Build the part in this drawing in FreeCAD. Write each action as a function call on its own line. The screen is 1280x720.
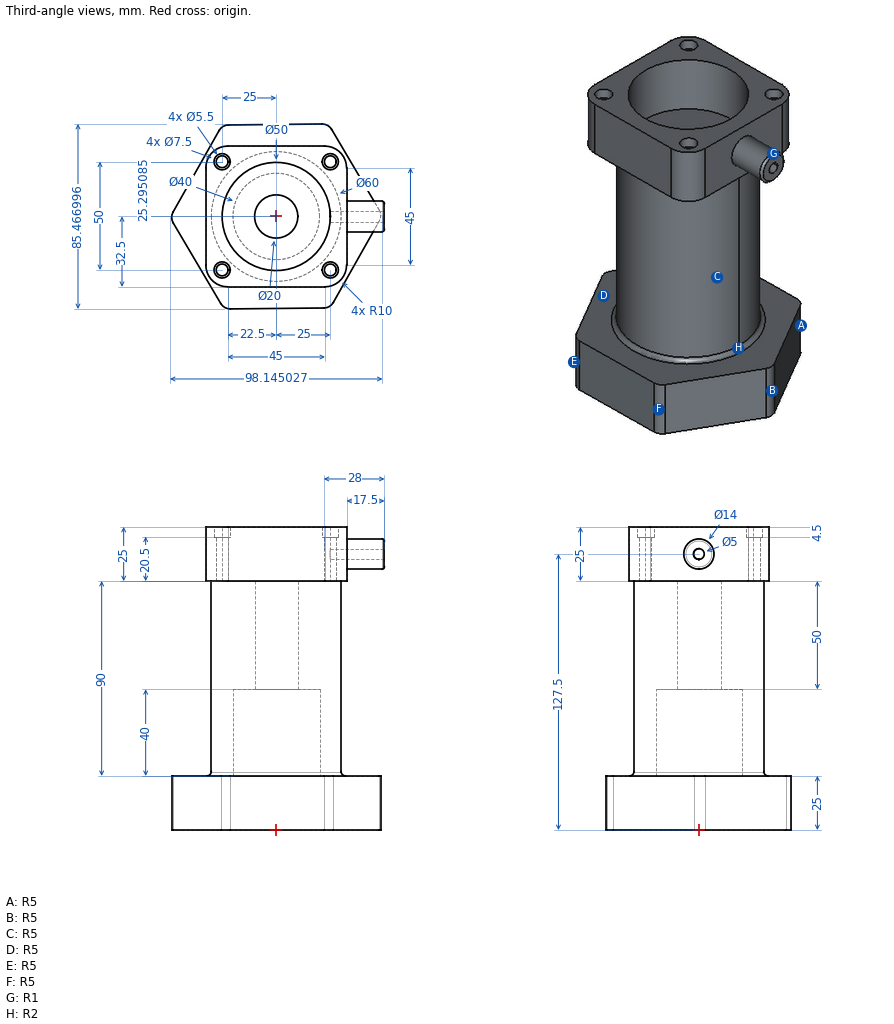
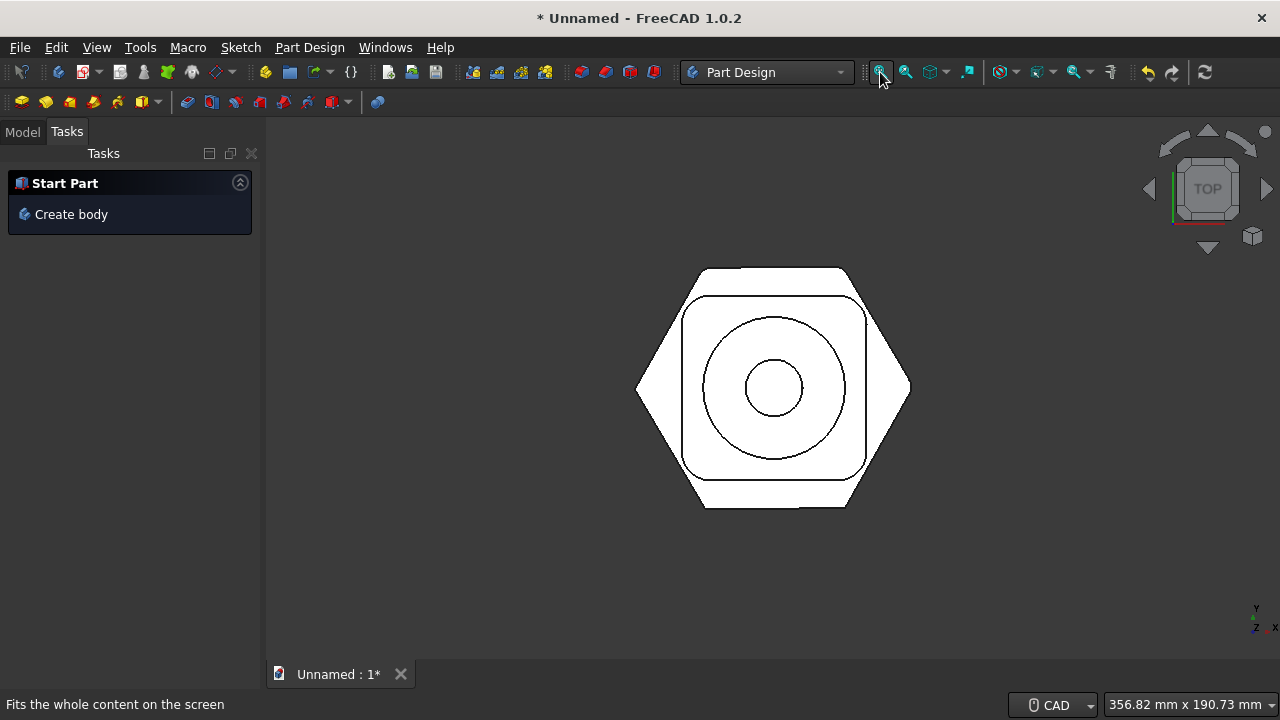
key(1)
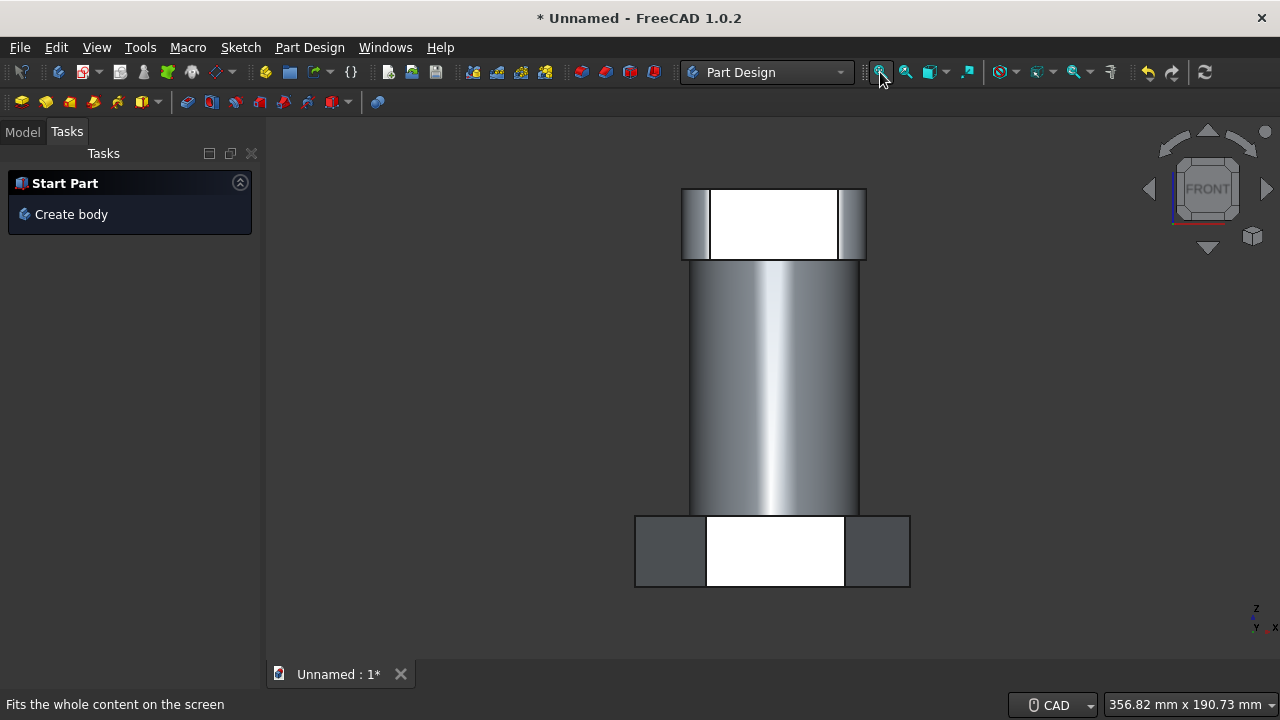
key(3)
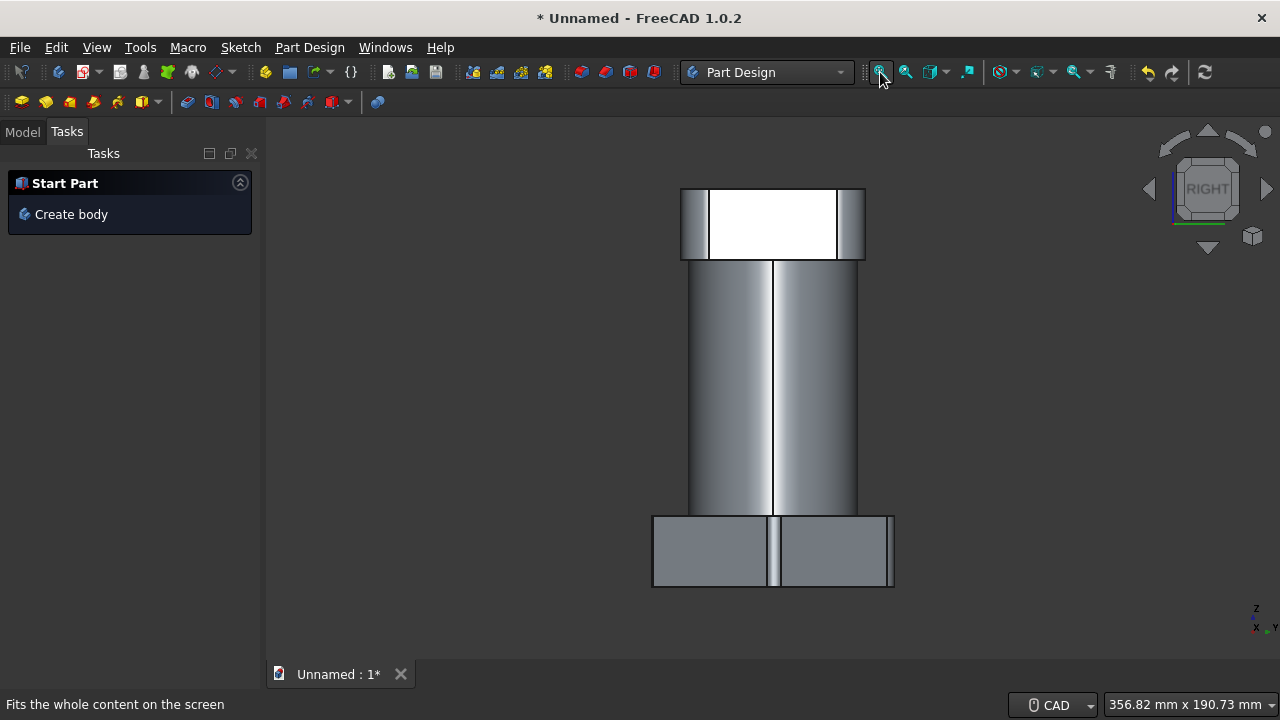
key(5)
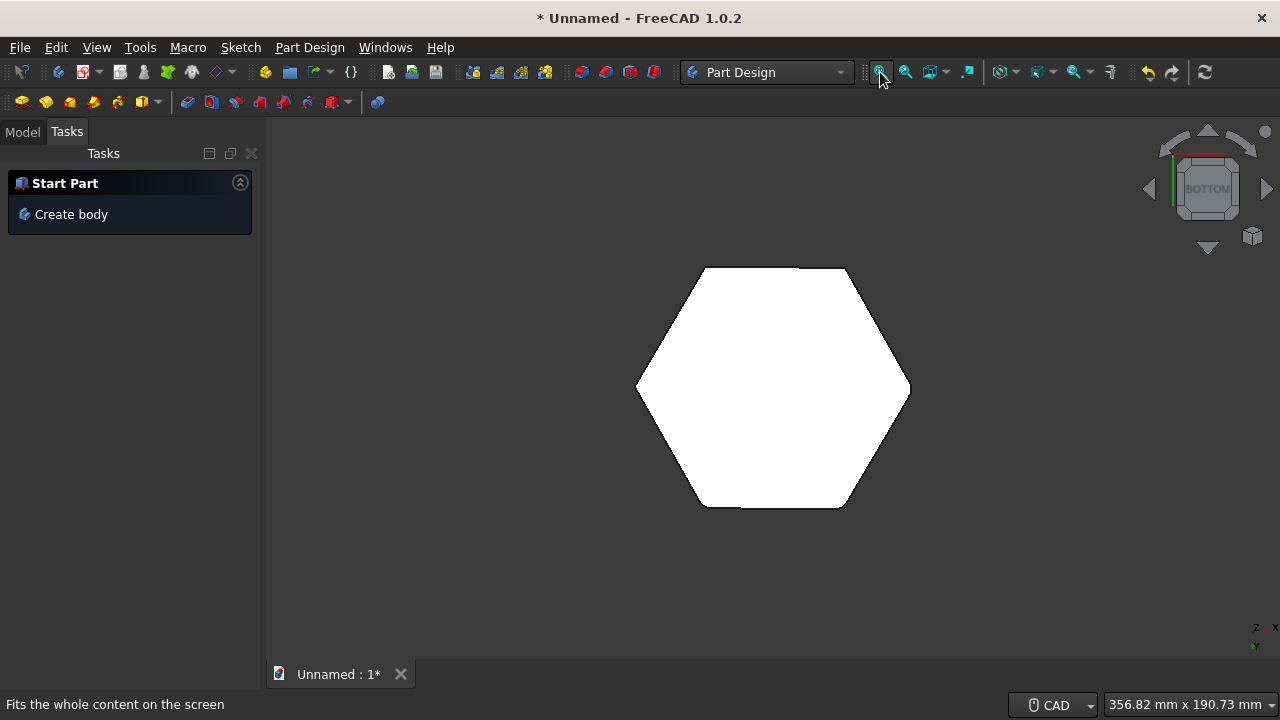
click(882, 72)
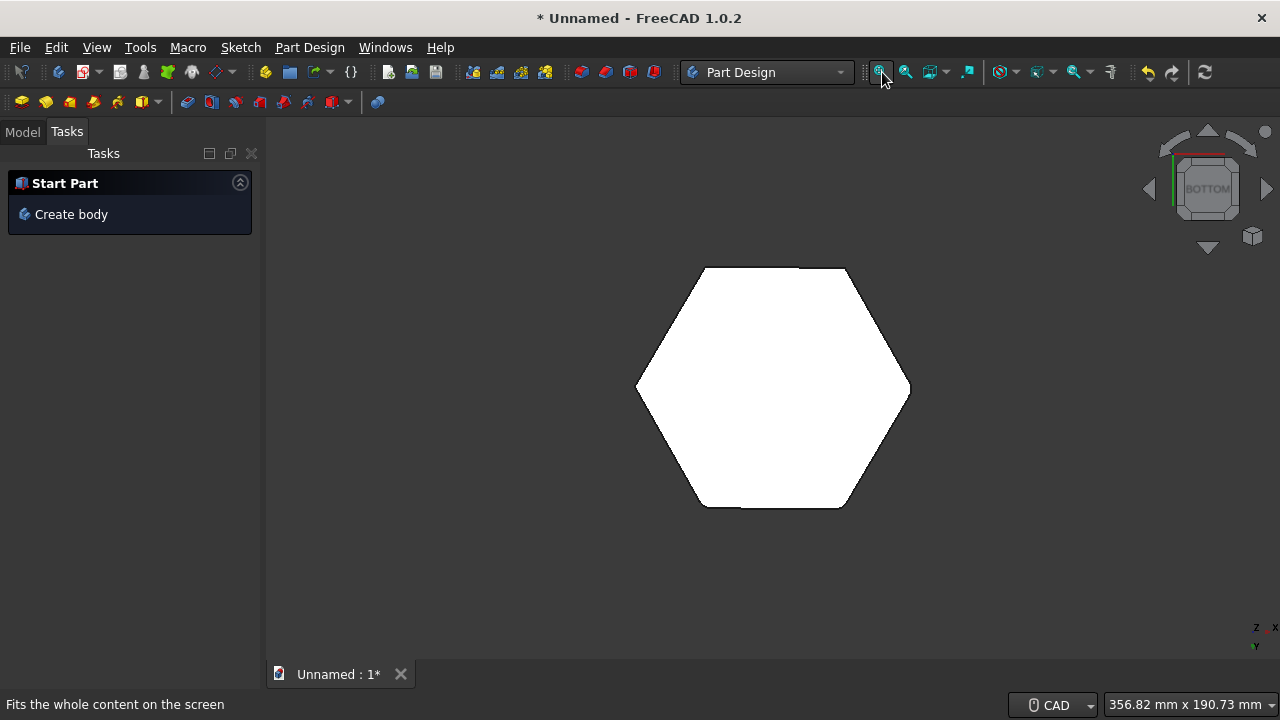
key(4)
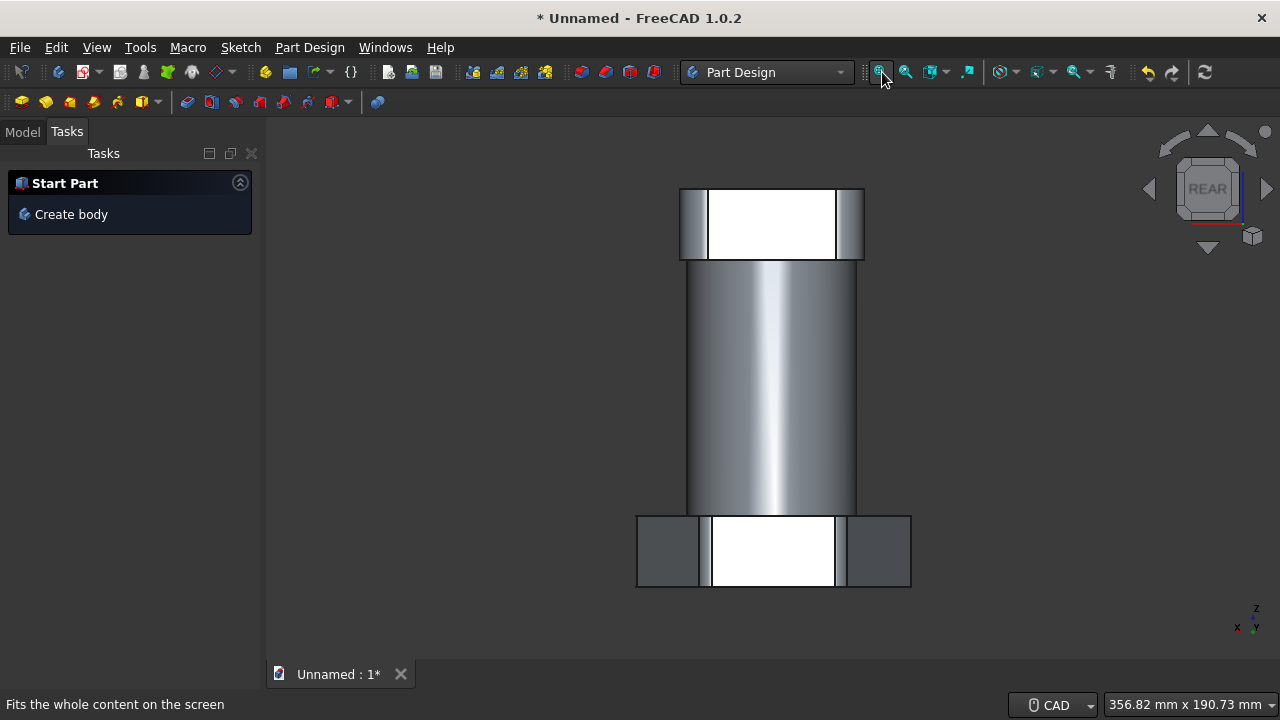
key(6)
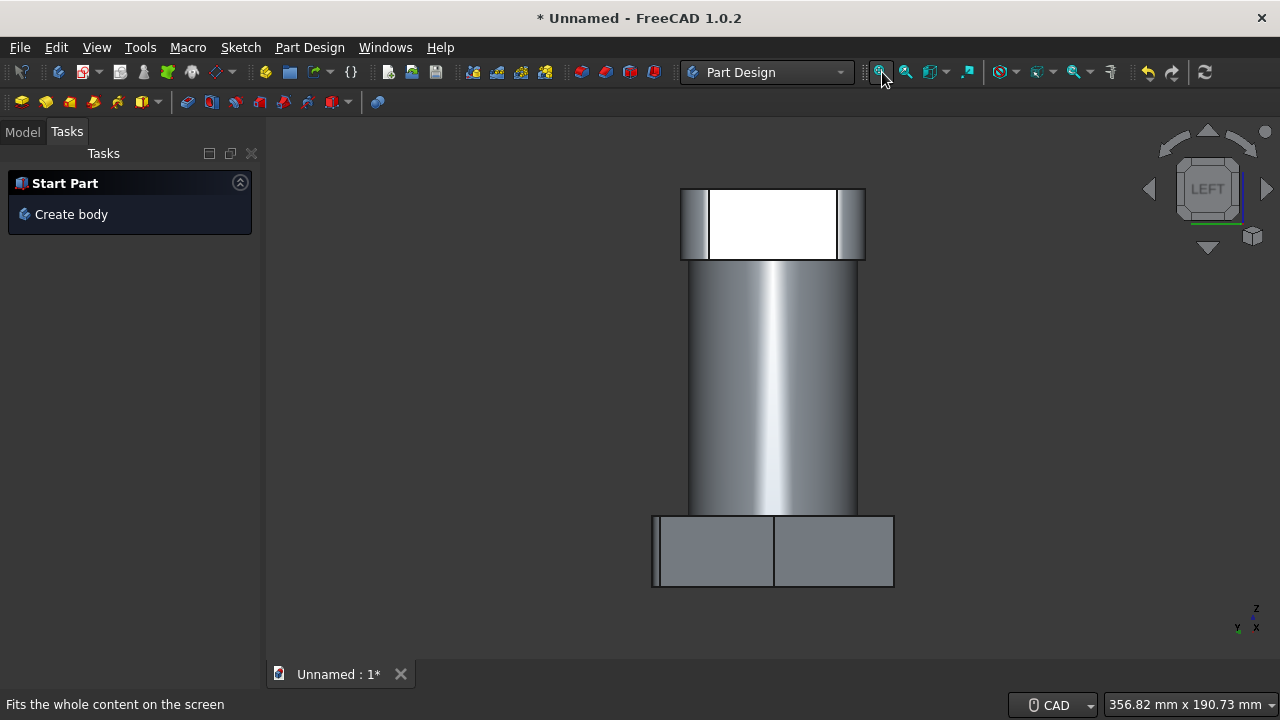
click(774, 550)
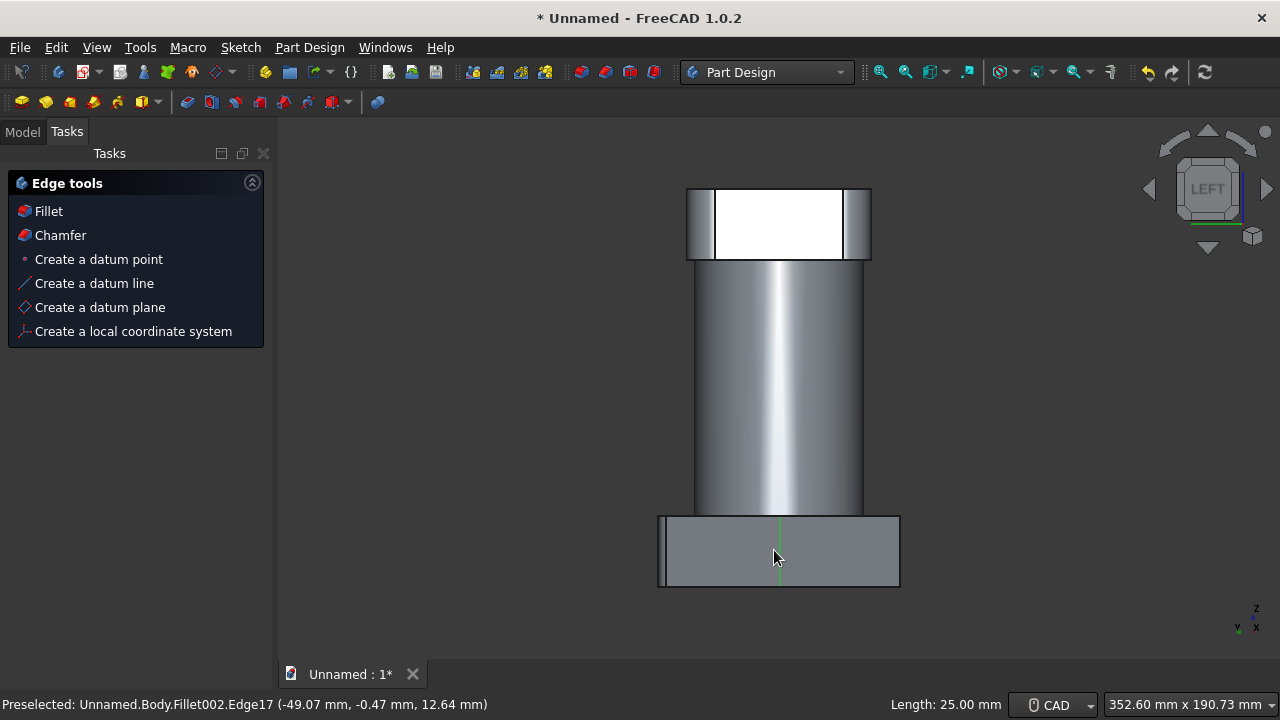
click(582, 72)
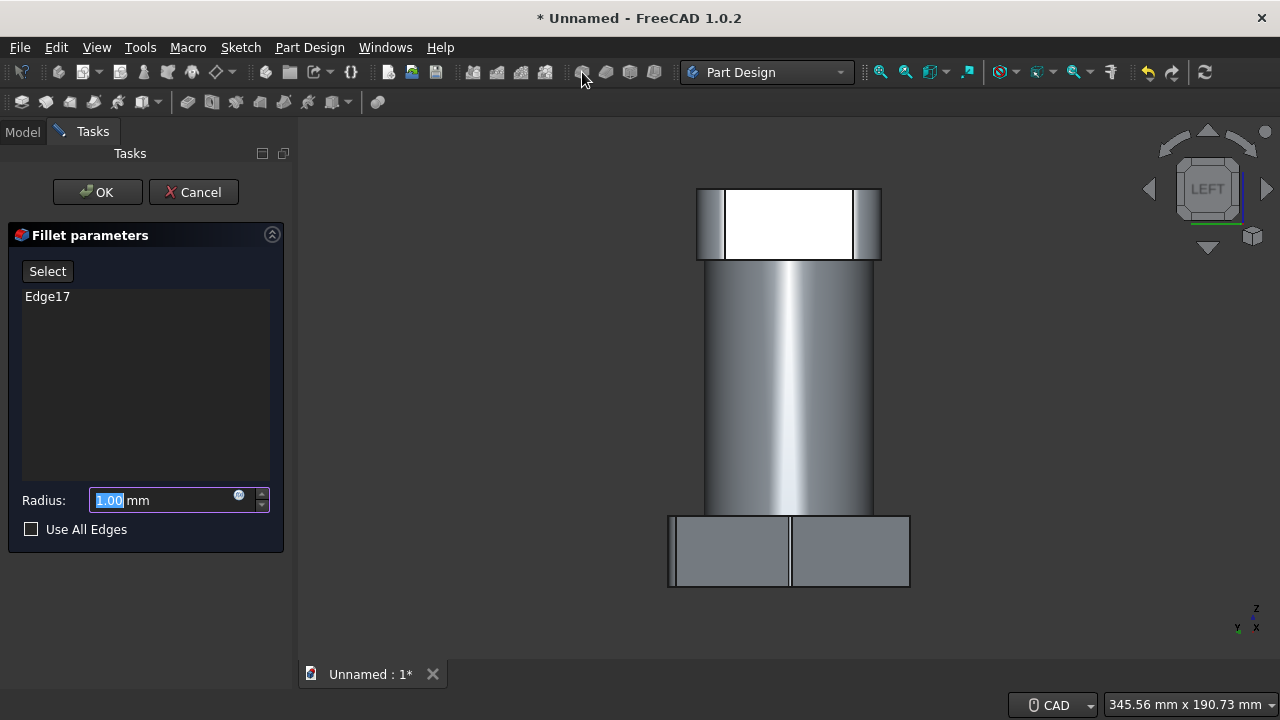
text(5)
key(Tab)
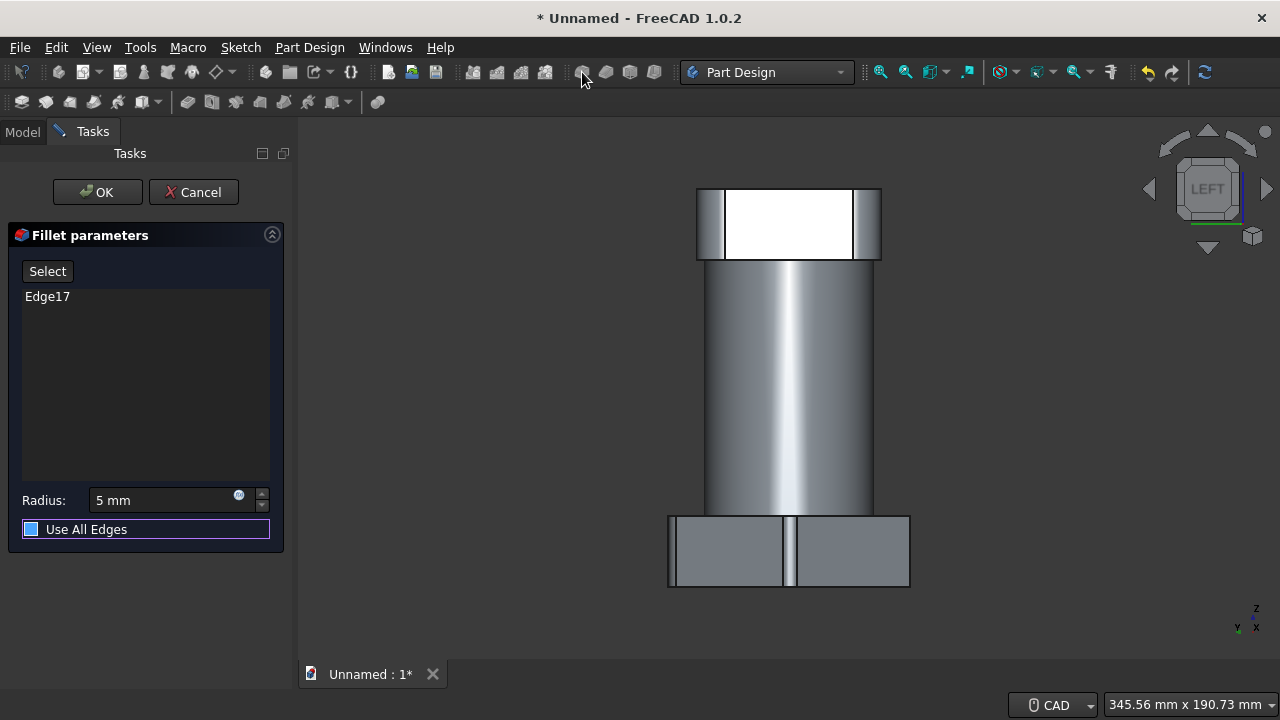
click(98, 192)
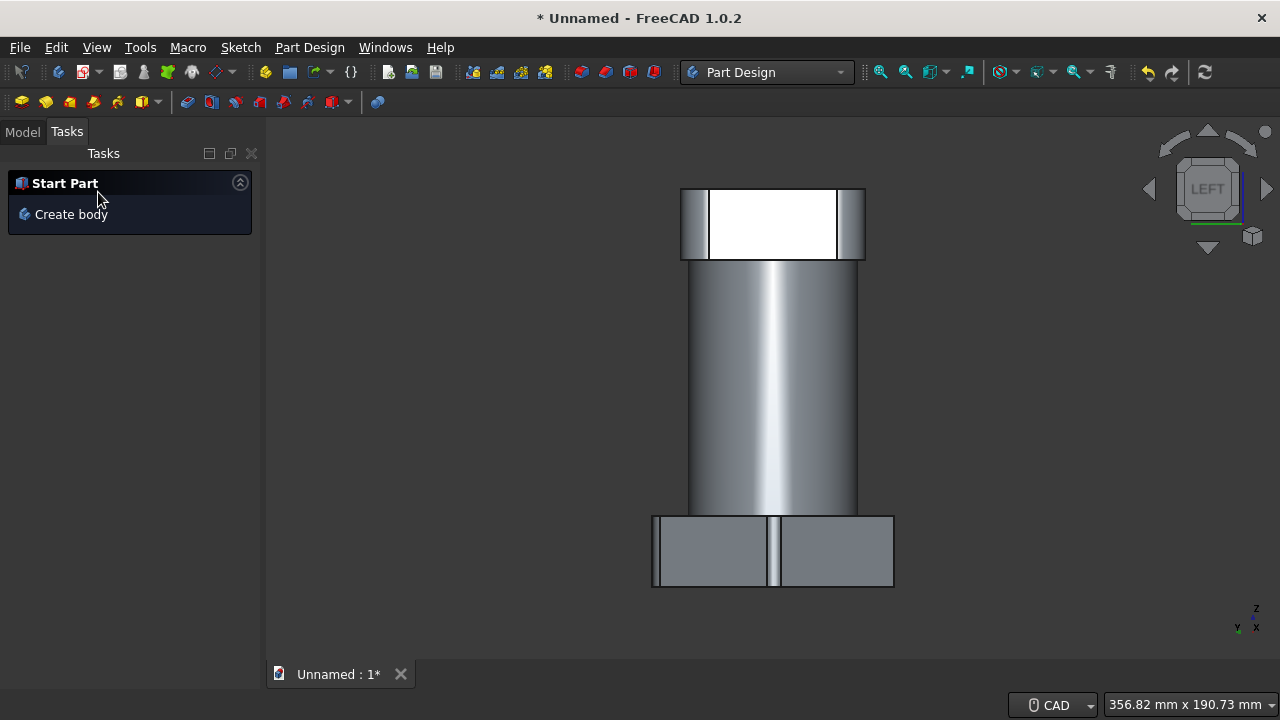
key(0)